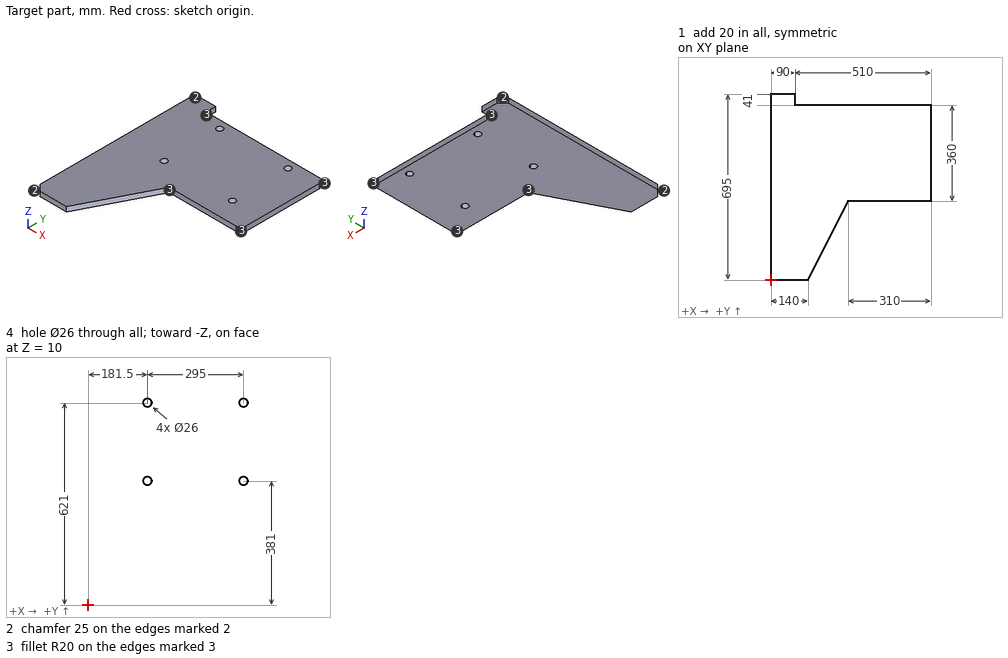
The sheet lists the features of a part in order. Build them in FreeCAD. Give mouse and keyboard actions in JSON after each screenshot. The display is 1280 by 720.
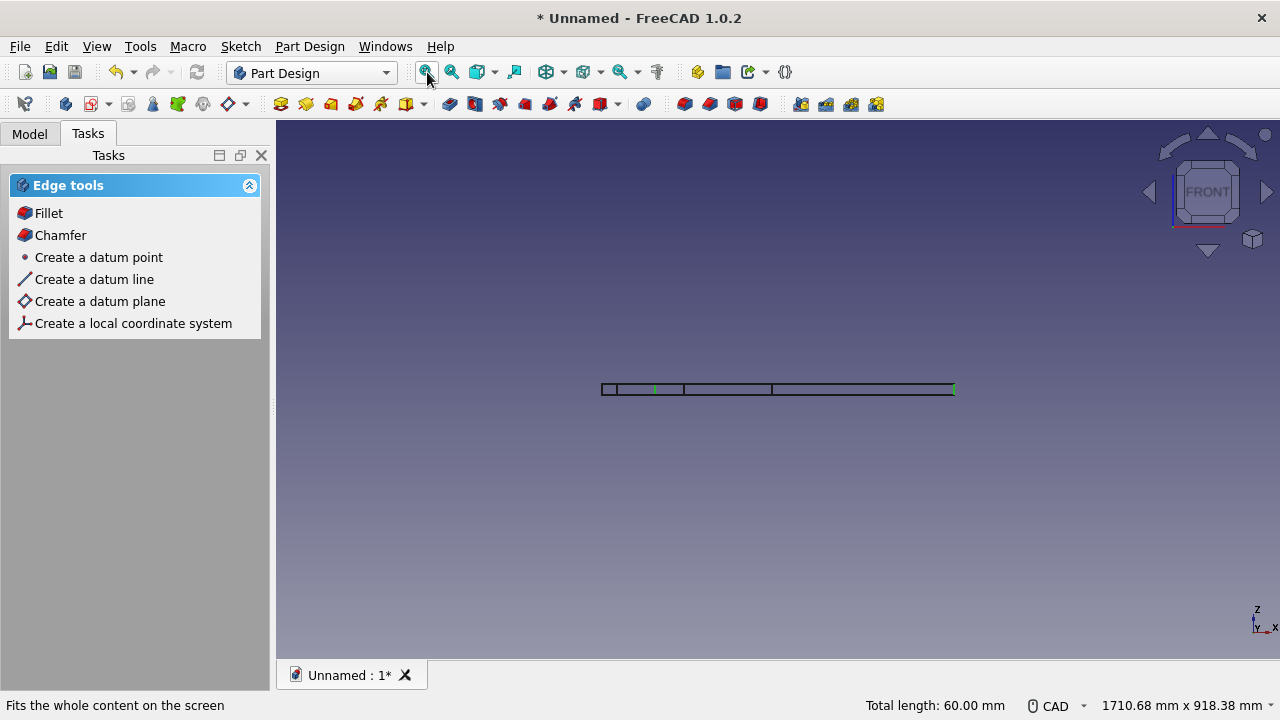
{"action": "scroll", "coordinate": [772, 389], "scroll_direction": "up", "scroll_amount": 7}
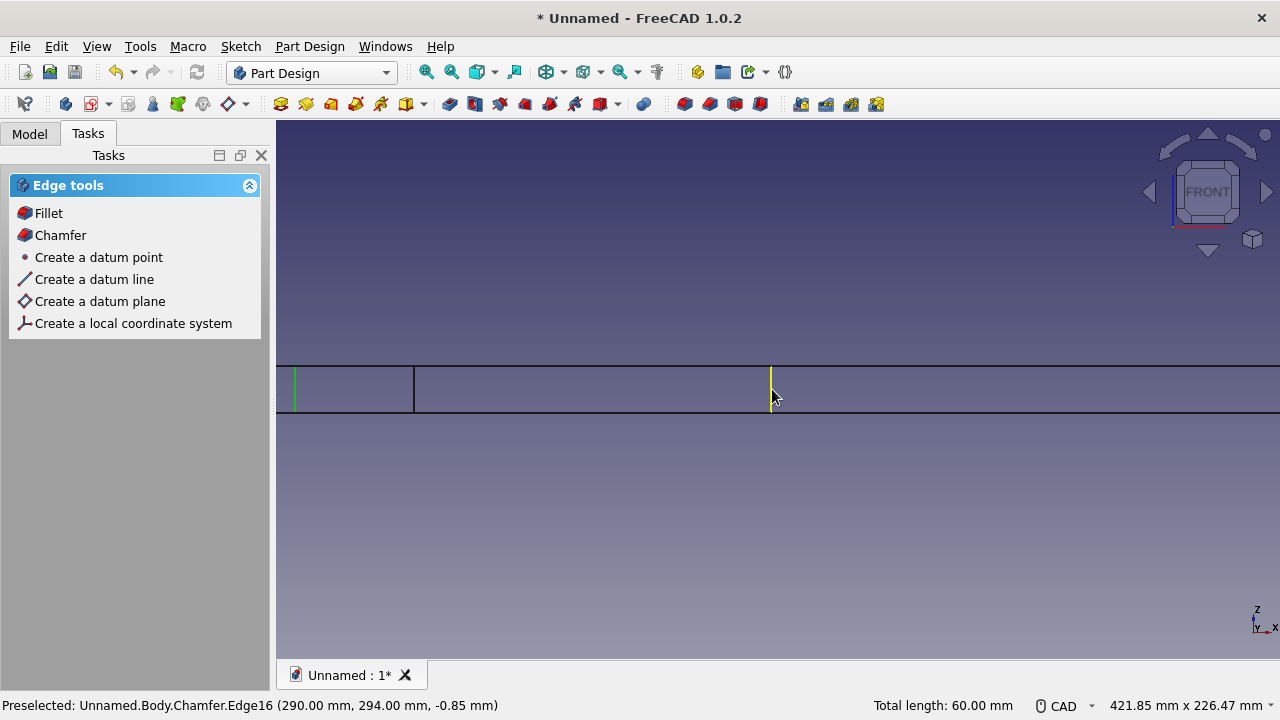
{"action": "left_click", "coordinate": [771, 389], "text": "ctrl"}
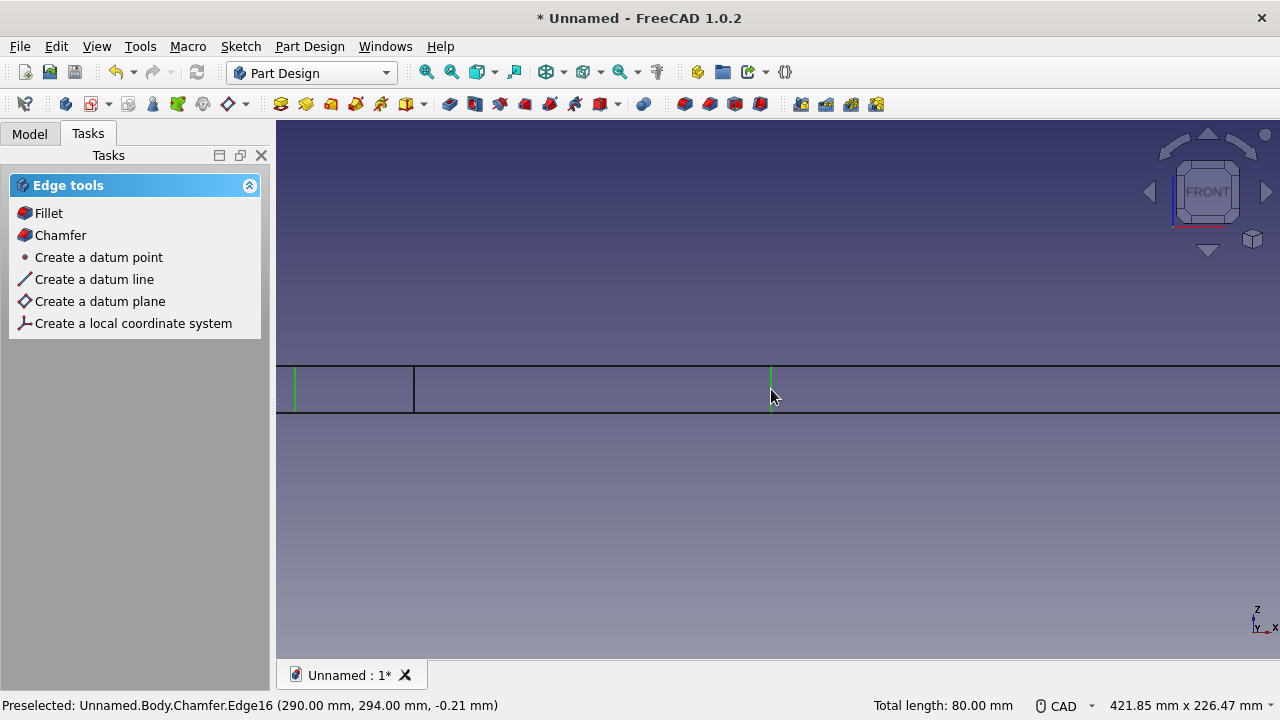
{"action": "key", "text": "v 1"}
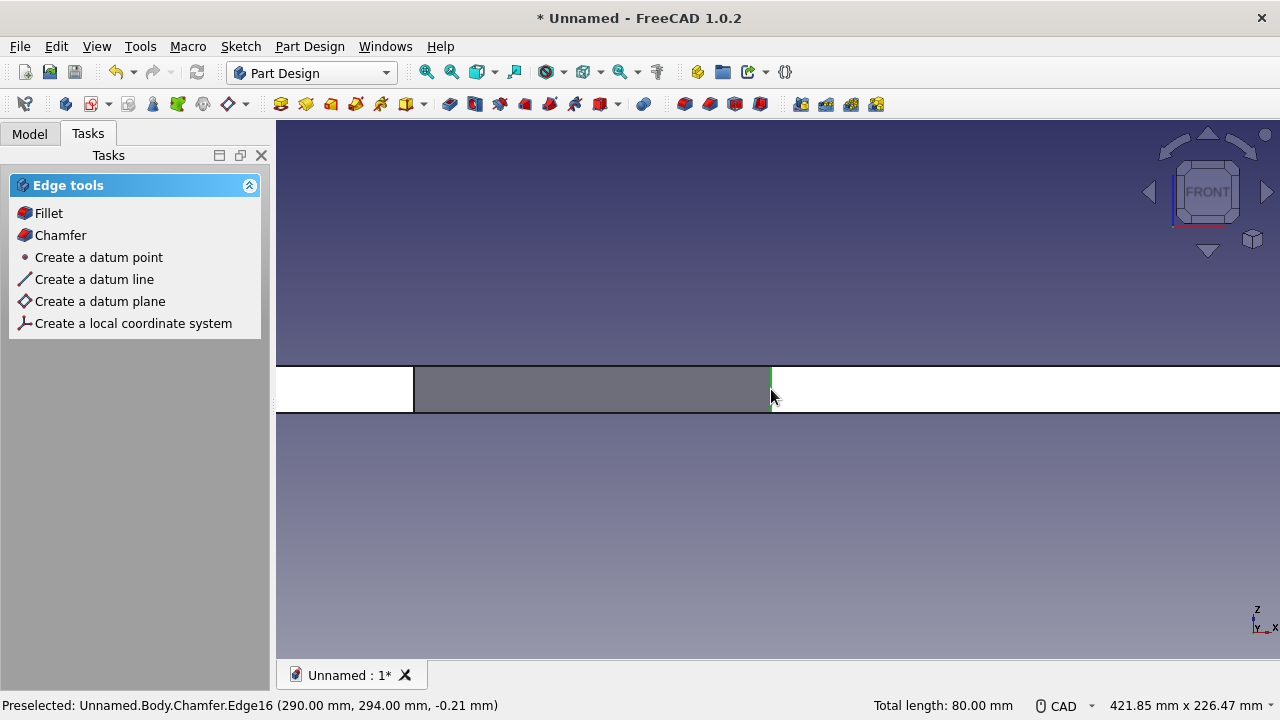
{"action": "left_click", "coordinate": [685, 104]}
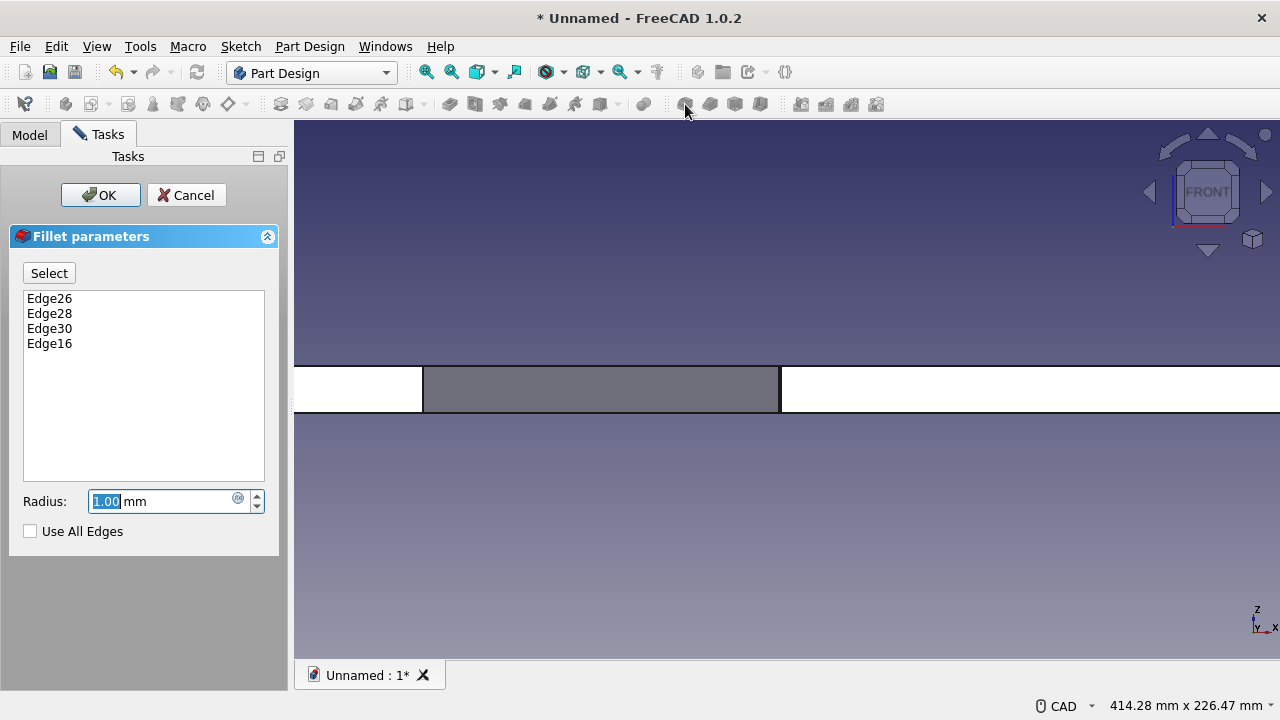
{"action": "type", "text": "20"}
{"action": "key", "text": "Tab"}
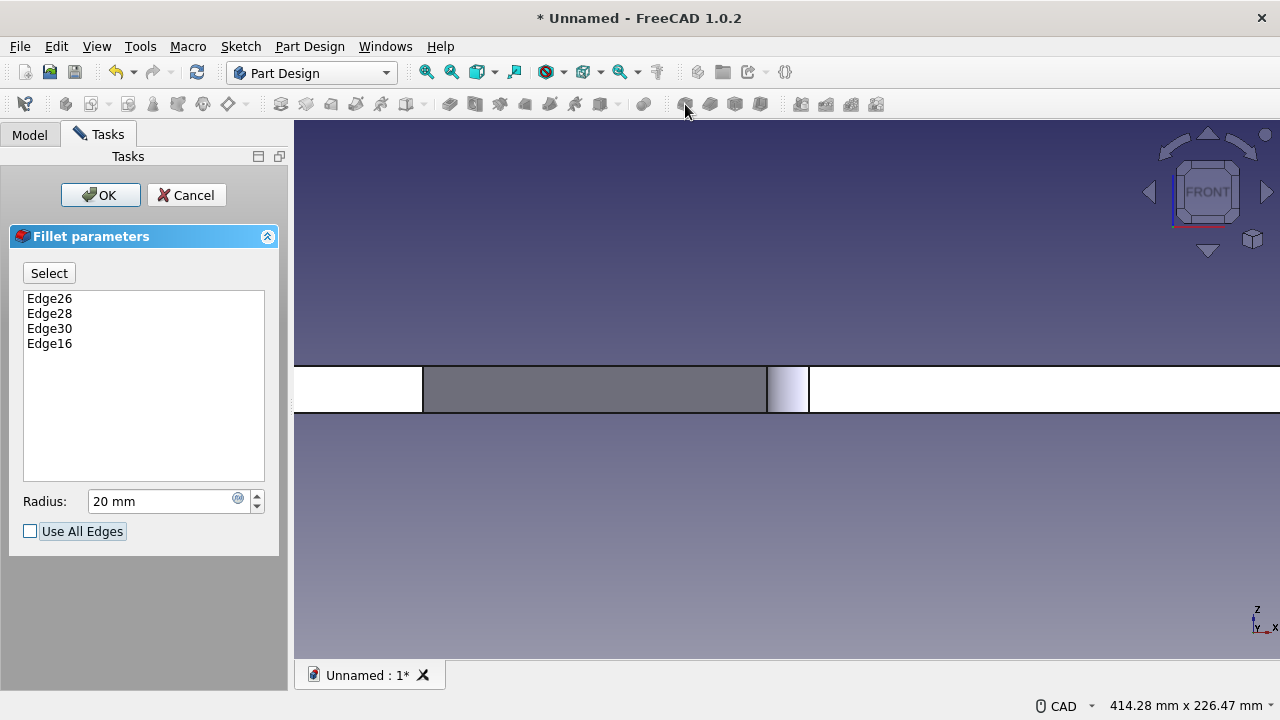
{"action": "left_click", "coordinate": [101, 195]}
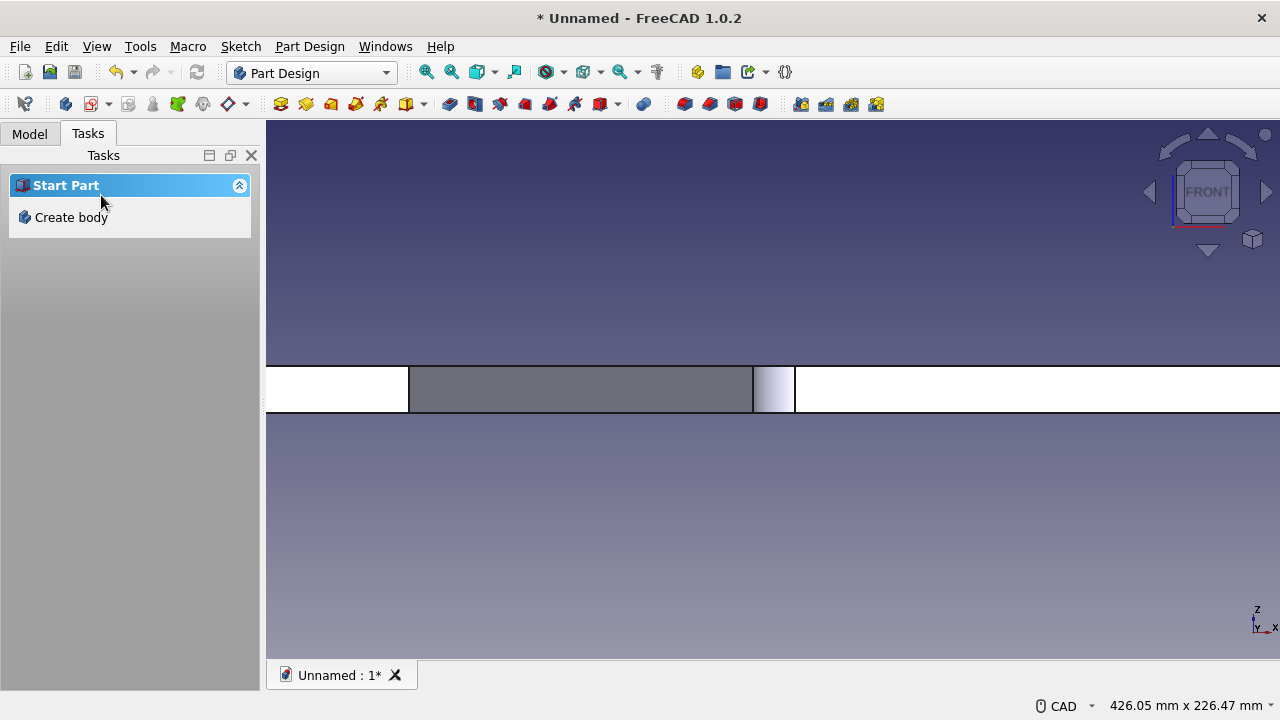
{"action": "left_click", "coordinate": [427, 72]}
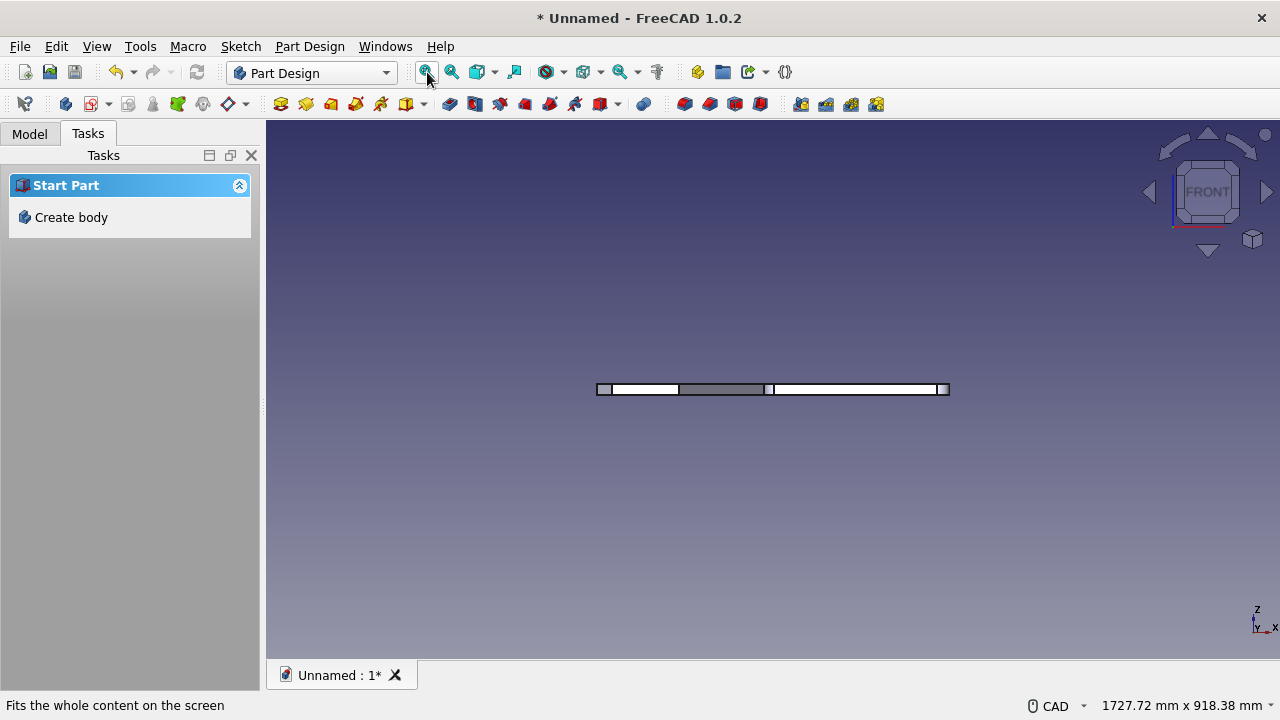
{"action": "key", "text": "0"}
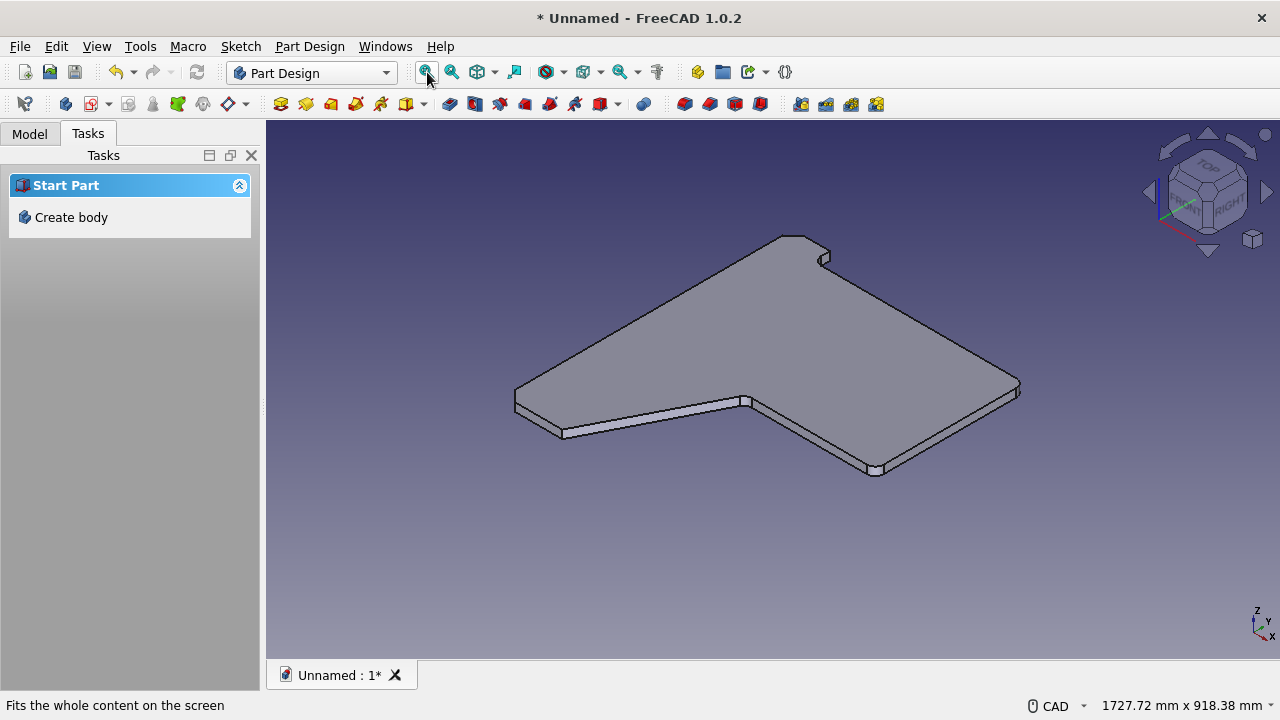
{"action": "left_click", "coordinate": [779, 339]}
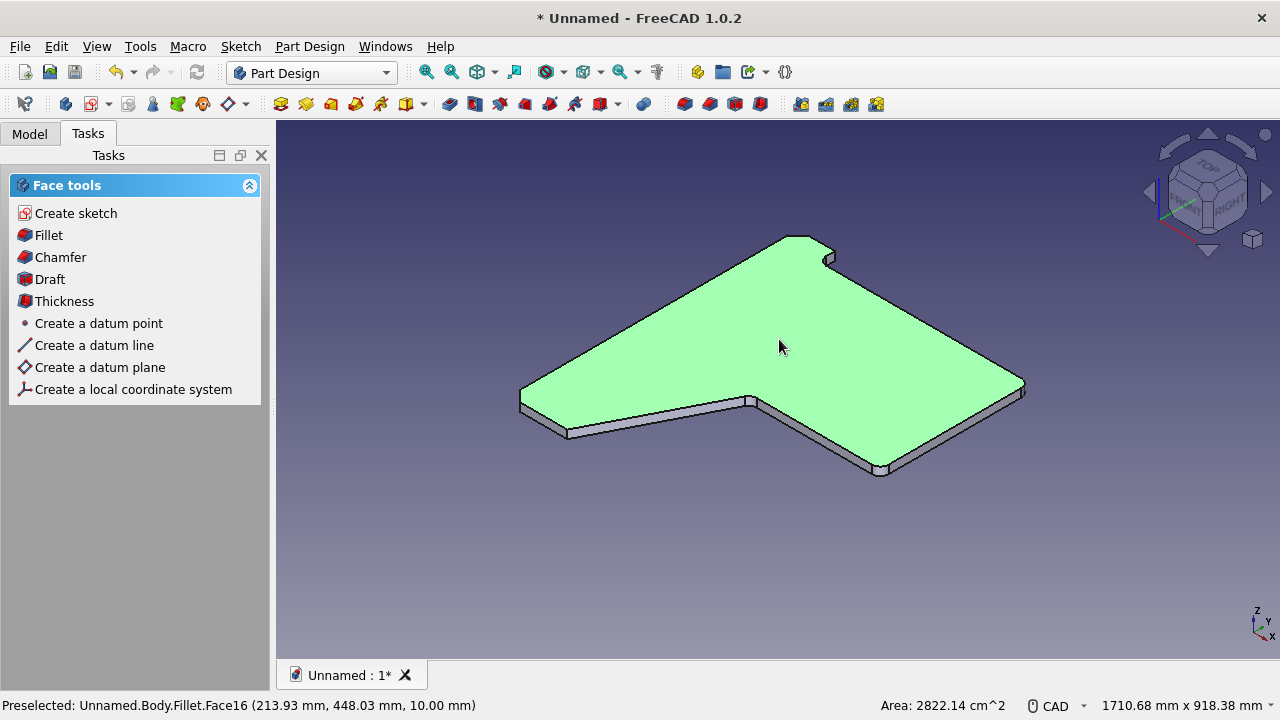
{"action": "left_click", "coordinate": [90, 104]}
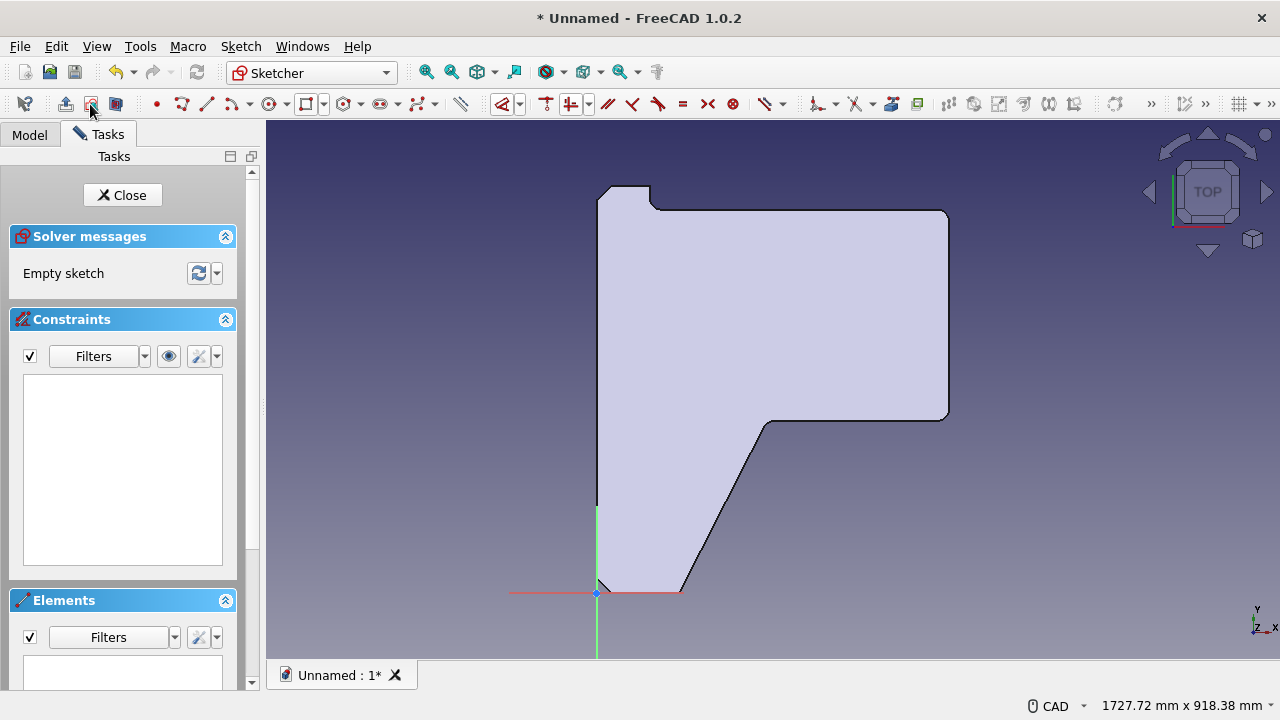
{"action": "left_click", "coordinate": [268, 104]}